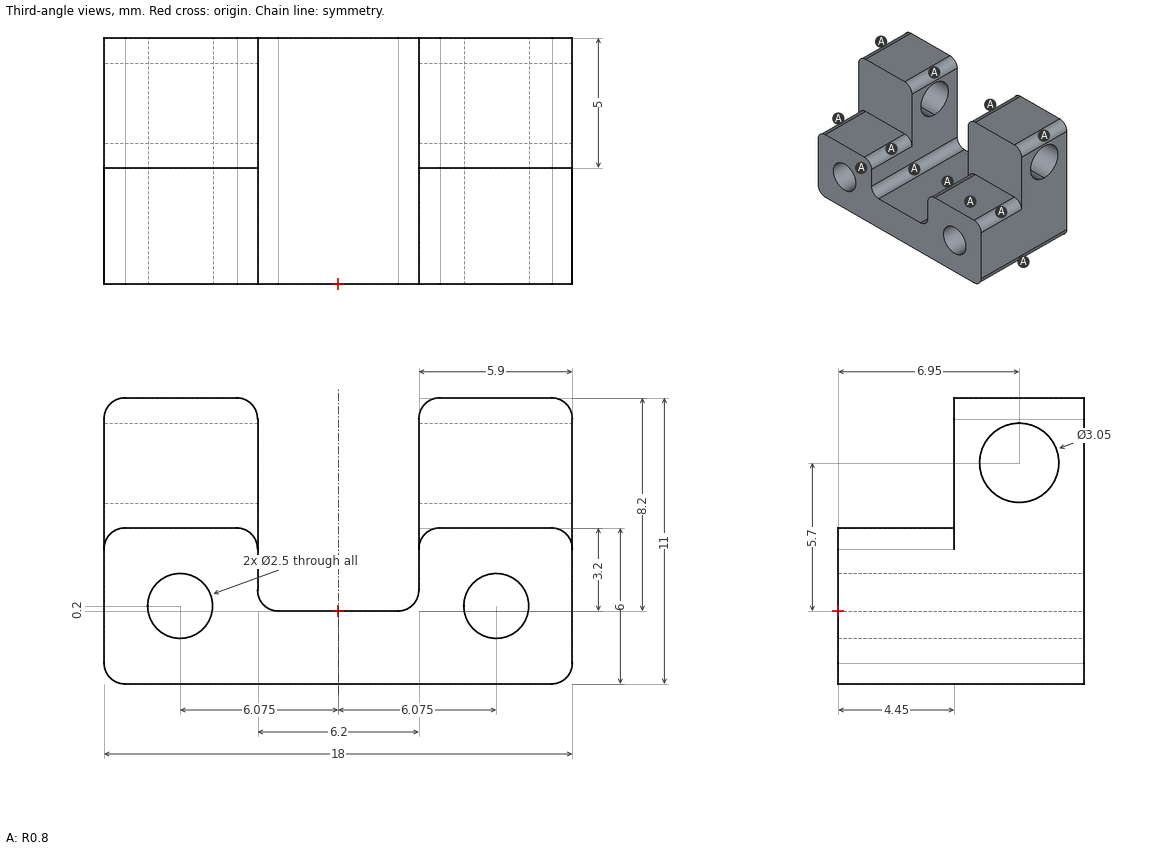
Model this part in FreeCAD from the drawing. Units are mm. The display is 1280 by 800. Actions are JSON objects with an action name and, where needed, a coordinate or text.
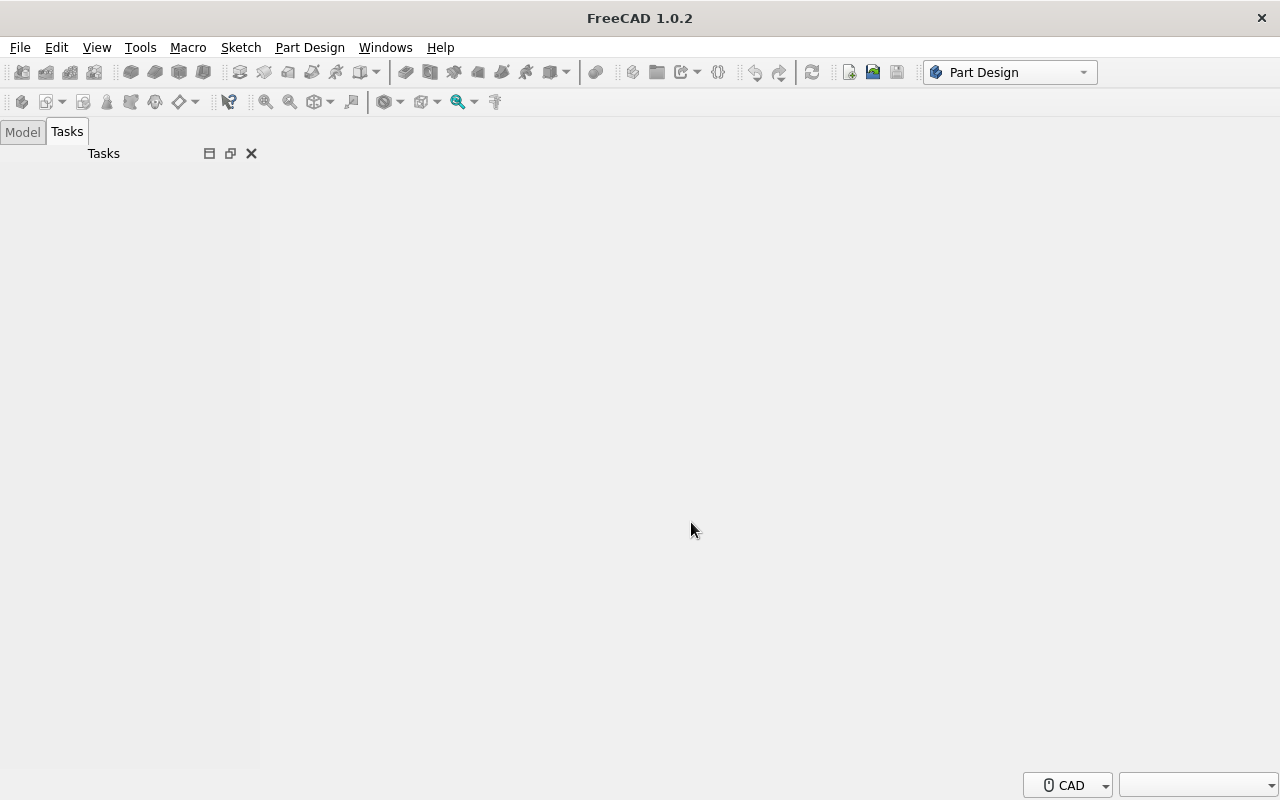
{"action": "left_click", "coordinate": [850, 72]}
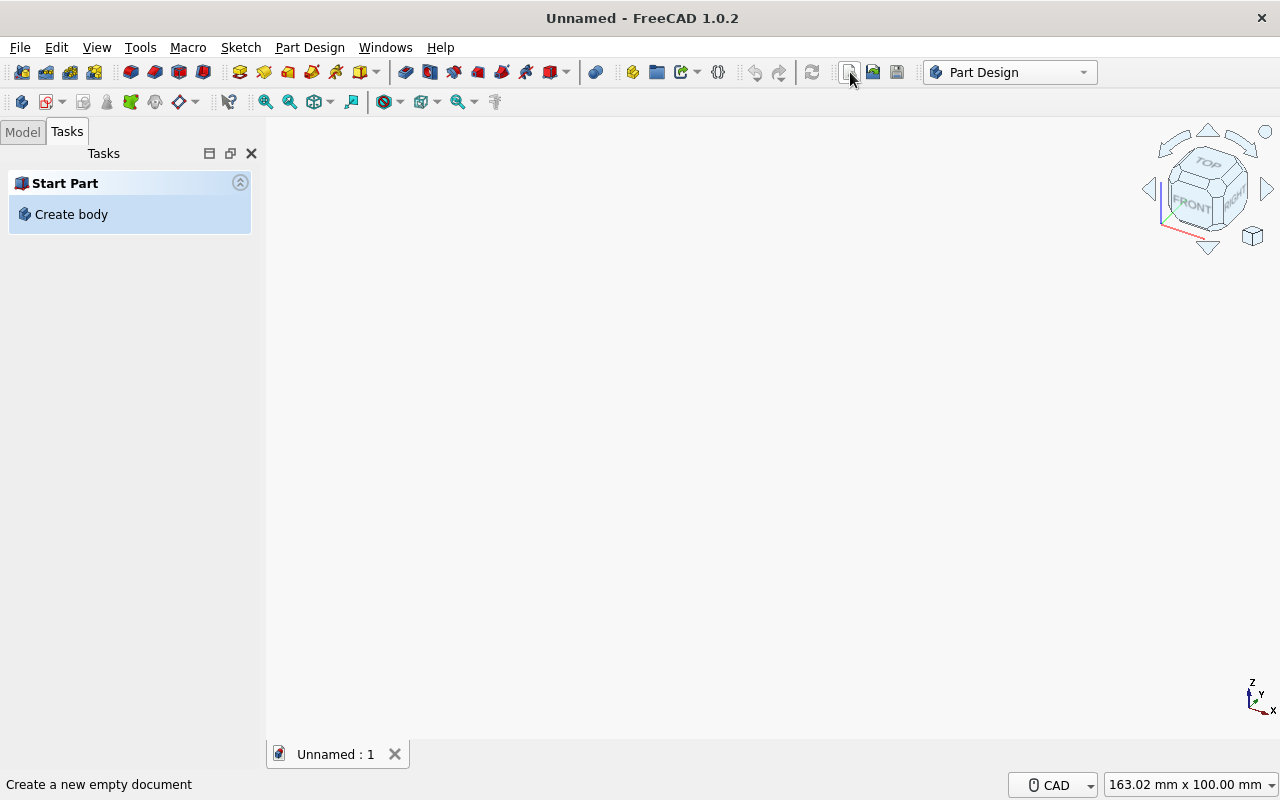
{"action": "left_click", "coordinate": [46, 102]}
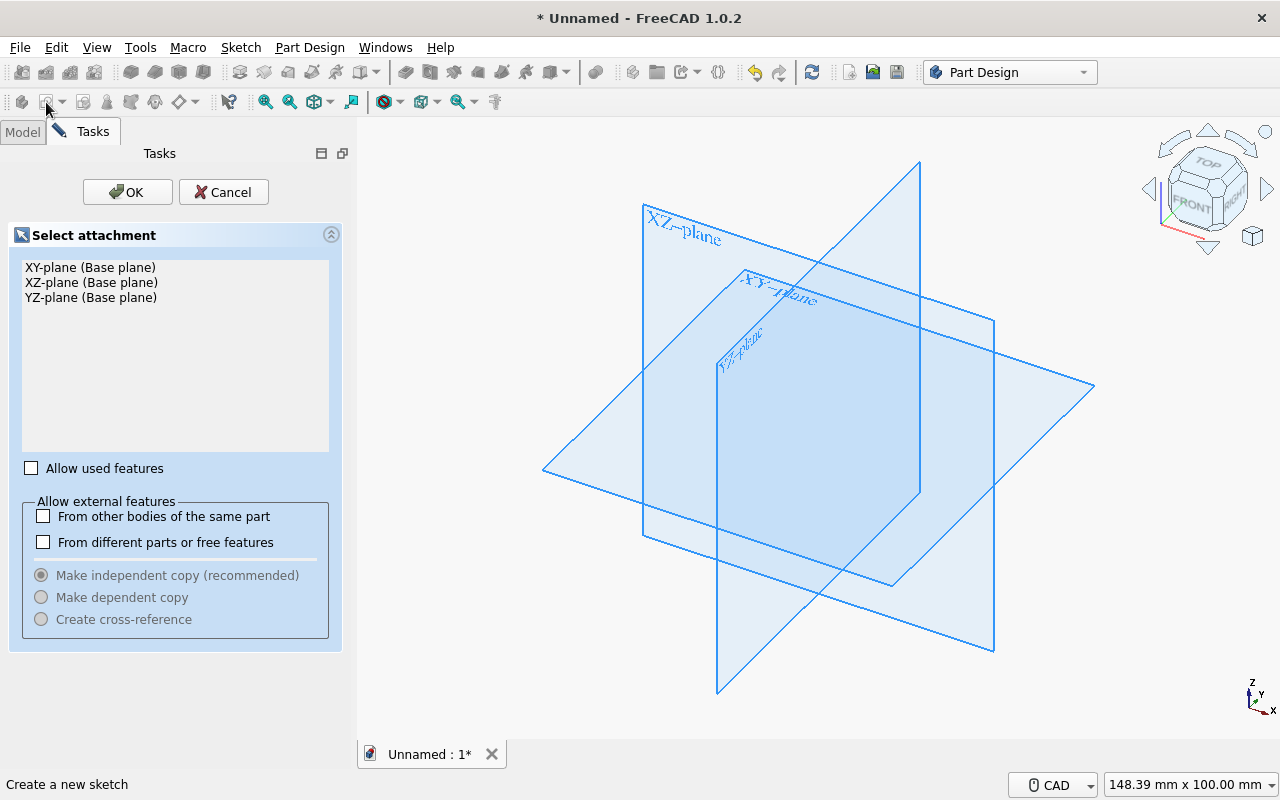
{"action": "left_click", "coordinate": [82, 282]}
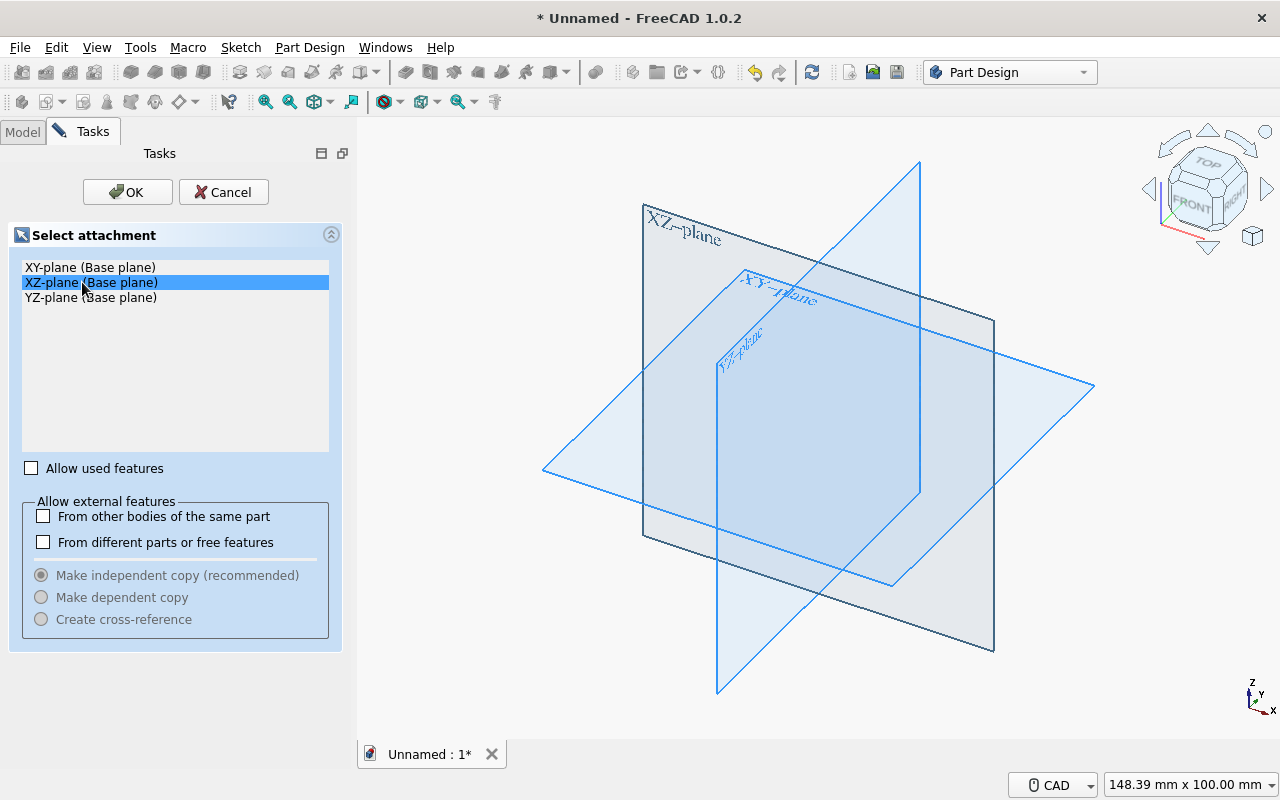
{"action": "left_click", "coordinate": [128, 192]}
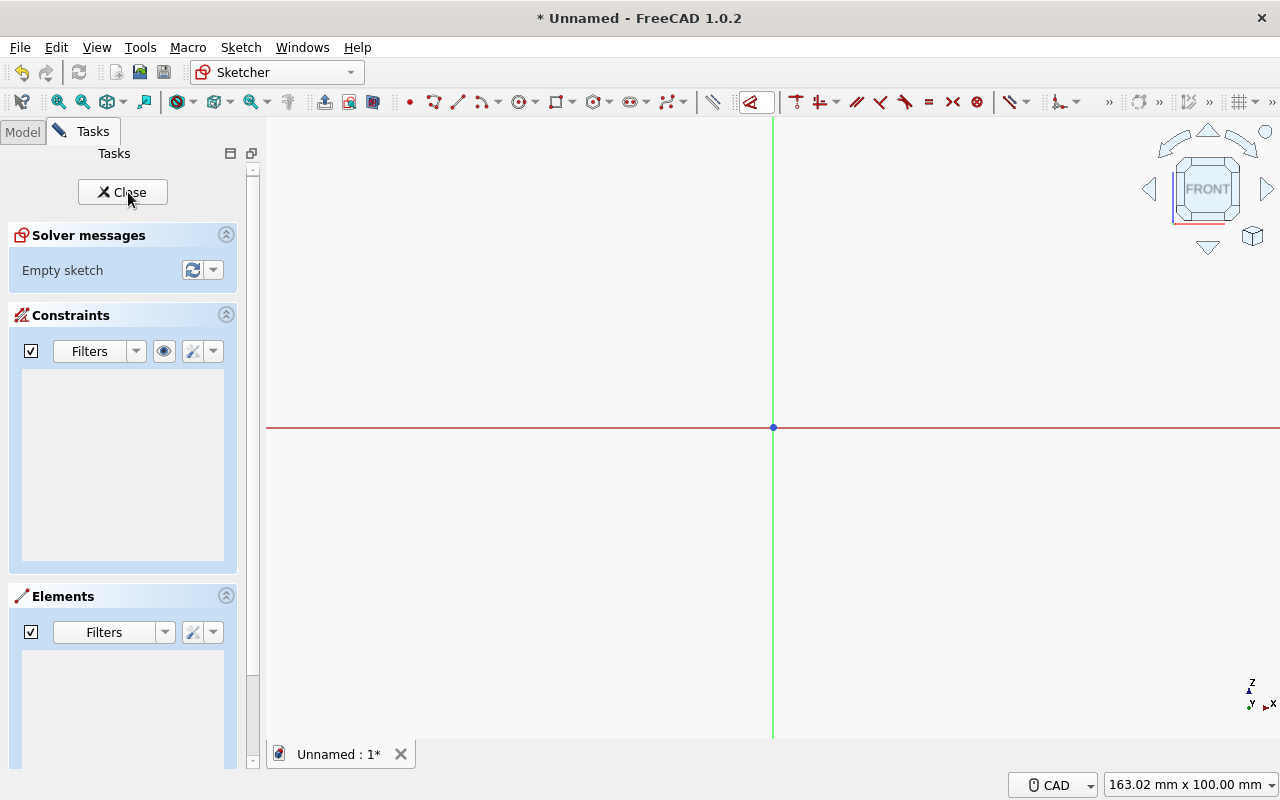
{"action": "scroll", "coordinate": [790, 426], "scroll_direction": "up", "scroll_amount": 8}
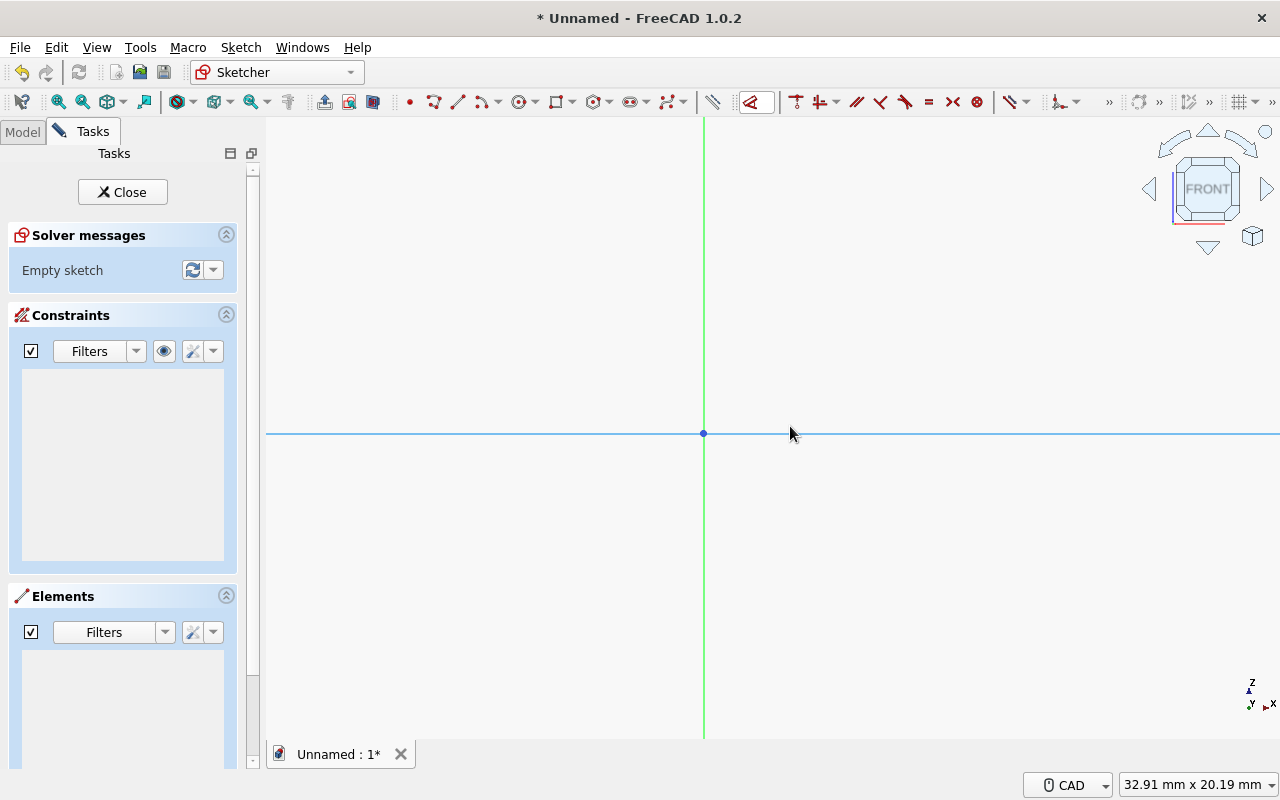
{"action": "left_click", "coordinate": [434, 102]}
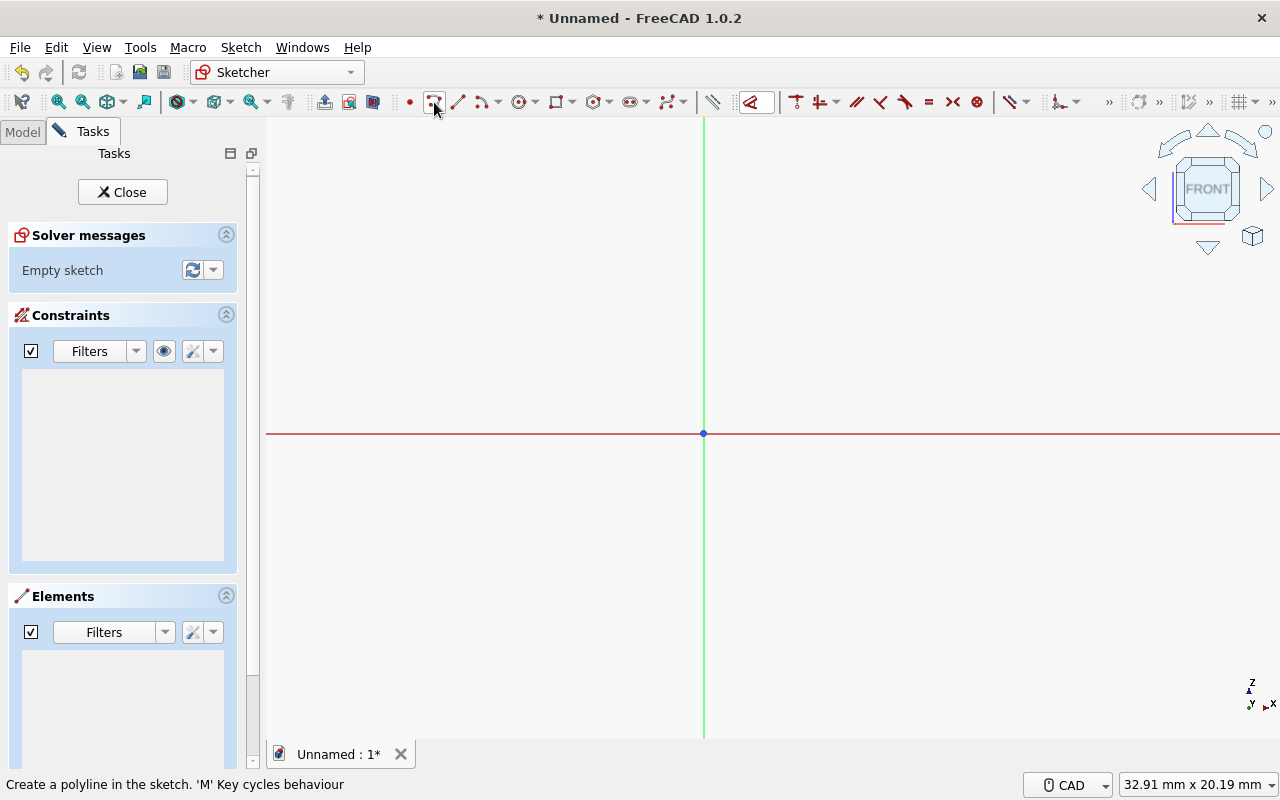
{"action": "left_click", "coordinate": [608, 434]}
{"action": "left_click", "coordinate": [799, 425]}
{"action": "left_click", "coordinate": [799, 335]}
{"action": "left_click", "coordinate": [981, 335]}
{"action": "left_click", "coordinate": [981, 520]}
{"action": "left_click", "coordinate": [426, 520]}
{"action": "left_click", "coordinate": [426, 335]}
{"action": "left_click", "coordinate": [608, 335]}
{"action": "left_click", "coordinate": [608, 434]}
{"action": "key", "text": "Escape"}
{"action": "key", "text": "Escape"}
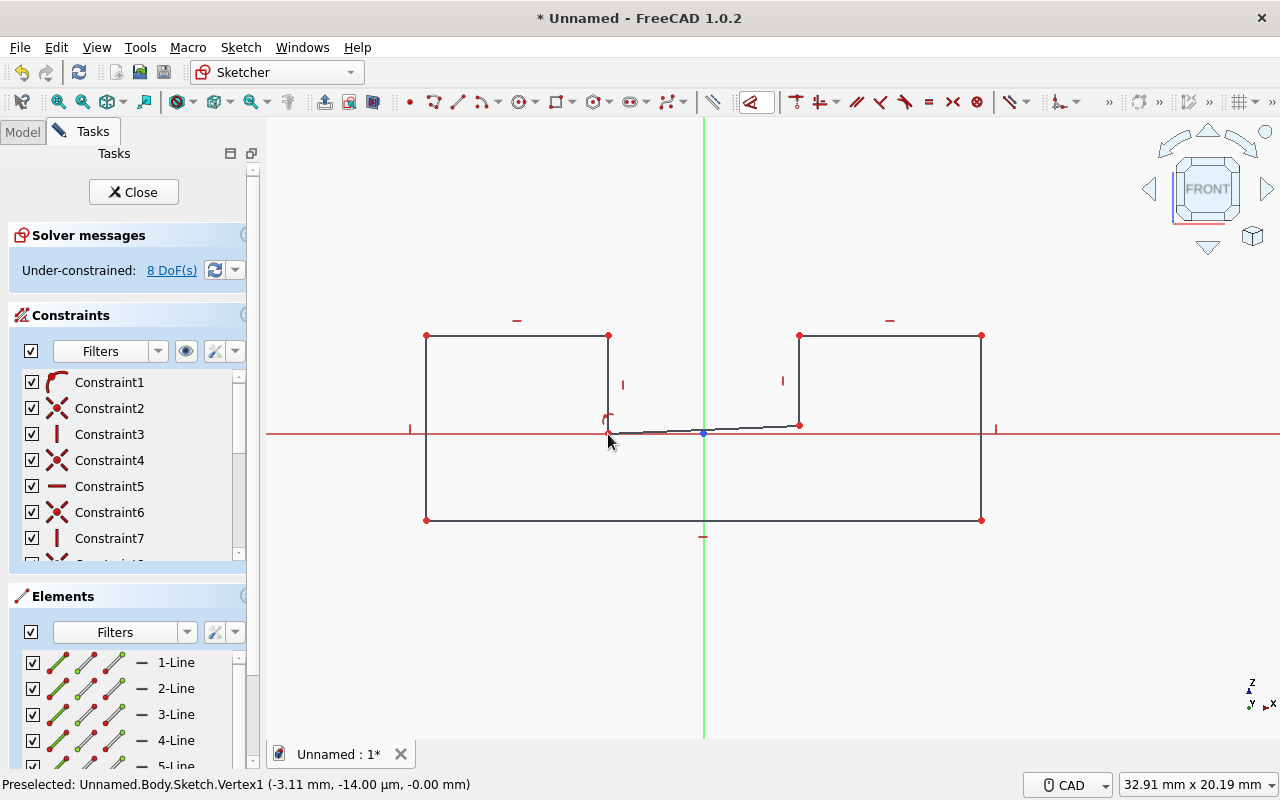
{"action": "left_click", "coordinate": [665, 432]}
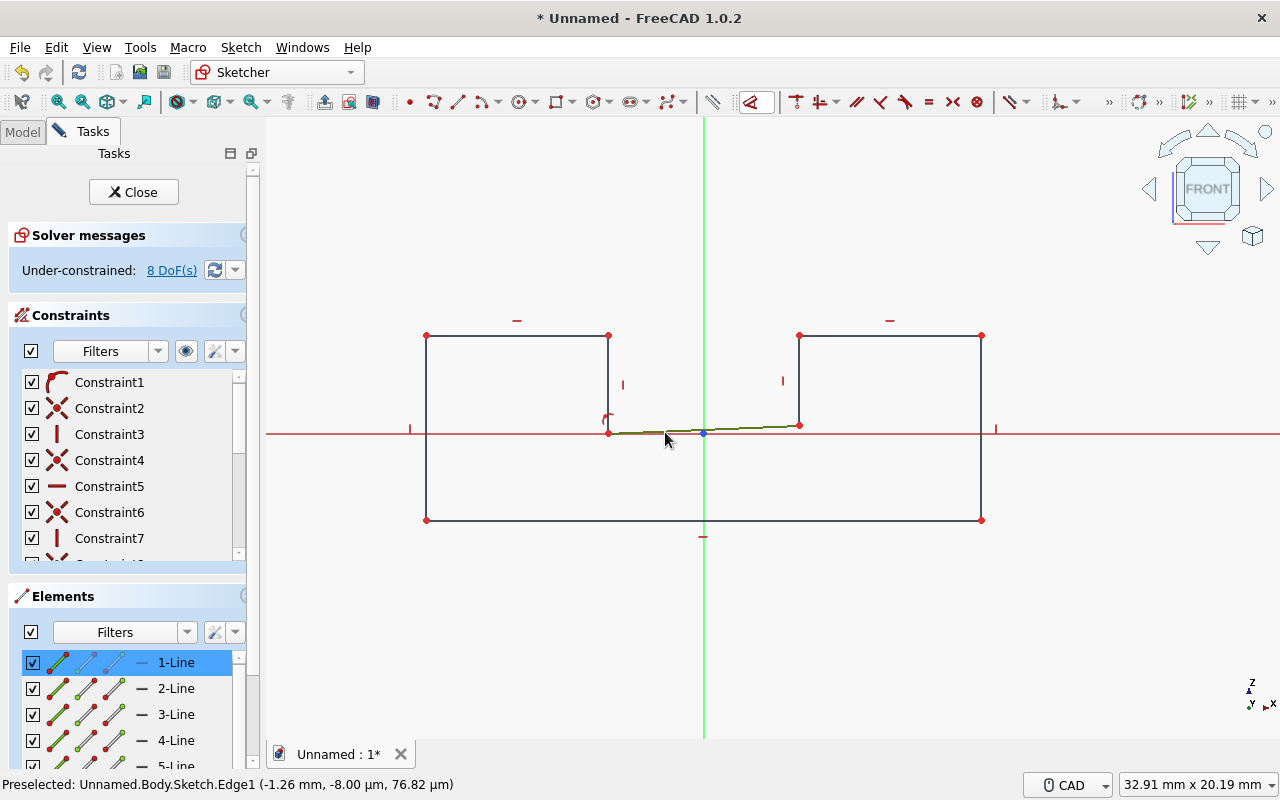
{"action": "key", "text": "h"}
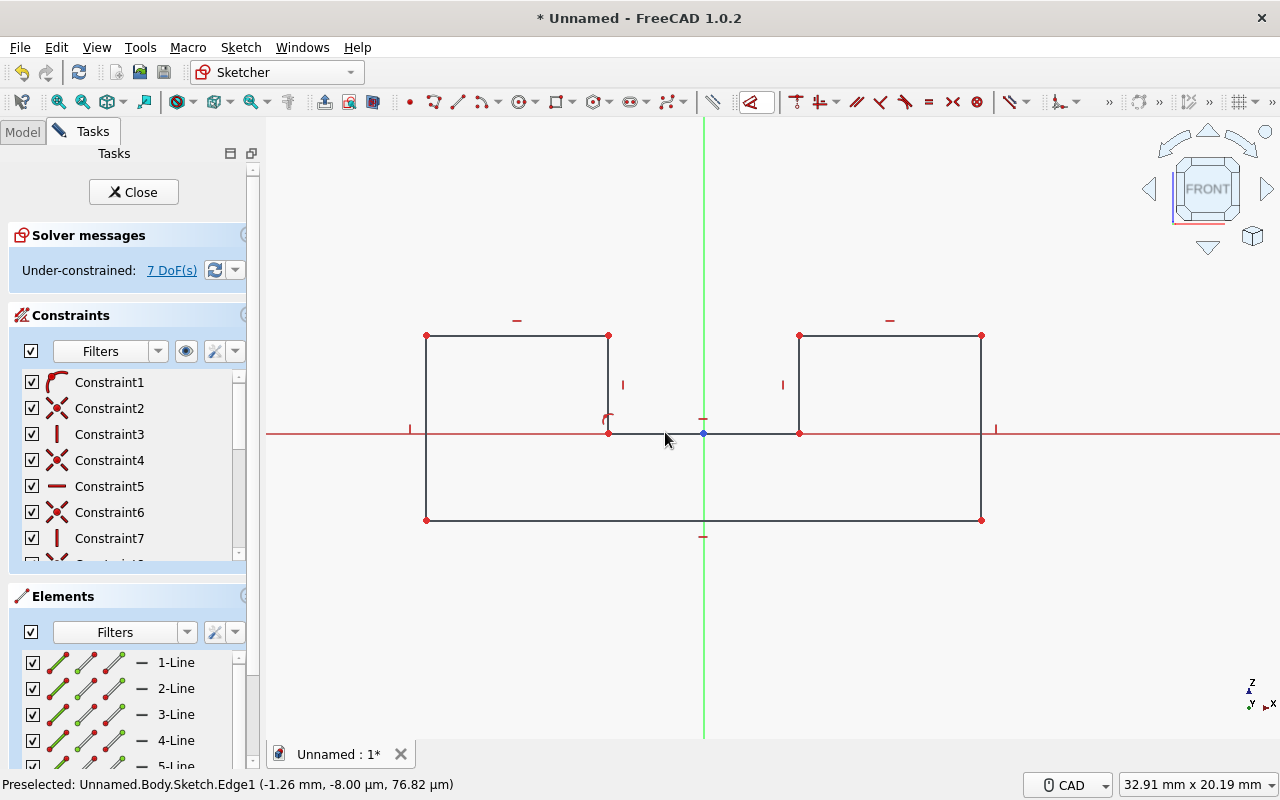
{"action": "left_click", "coordinate": [981, 336]}